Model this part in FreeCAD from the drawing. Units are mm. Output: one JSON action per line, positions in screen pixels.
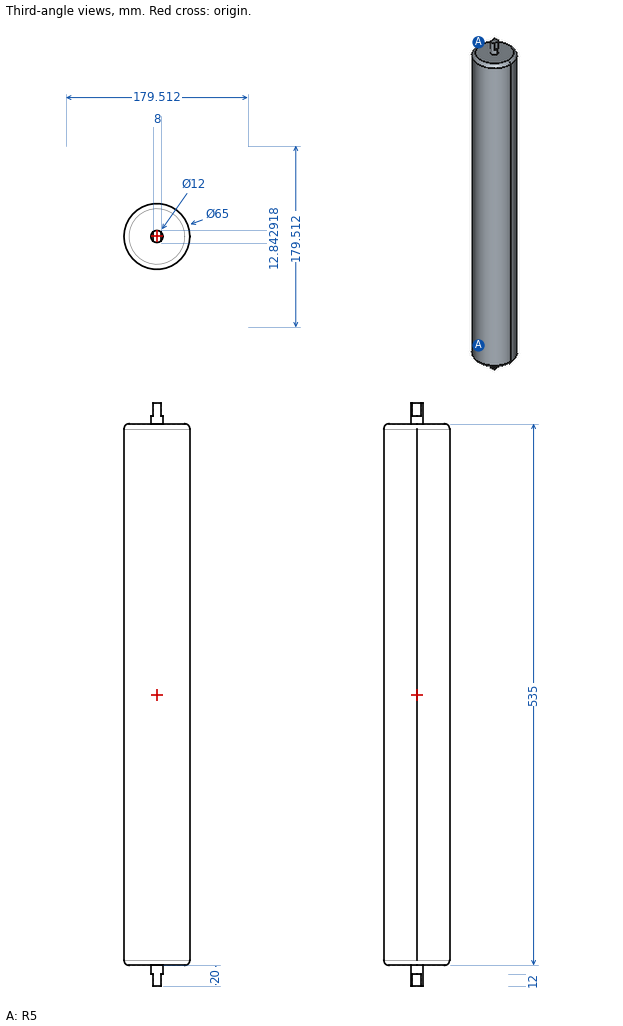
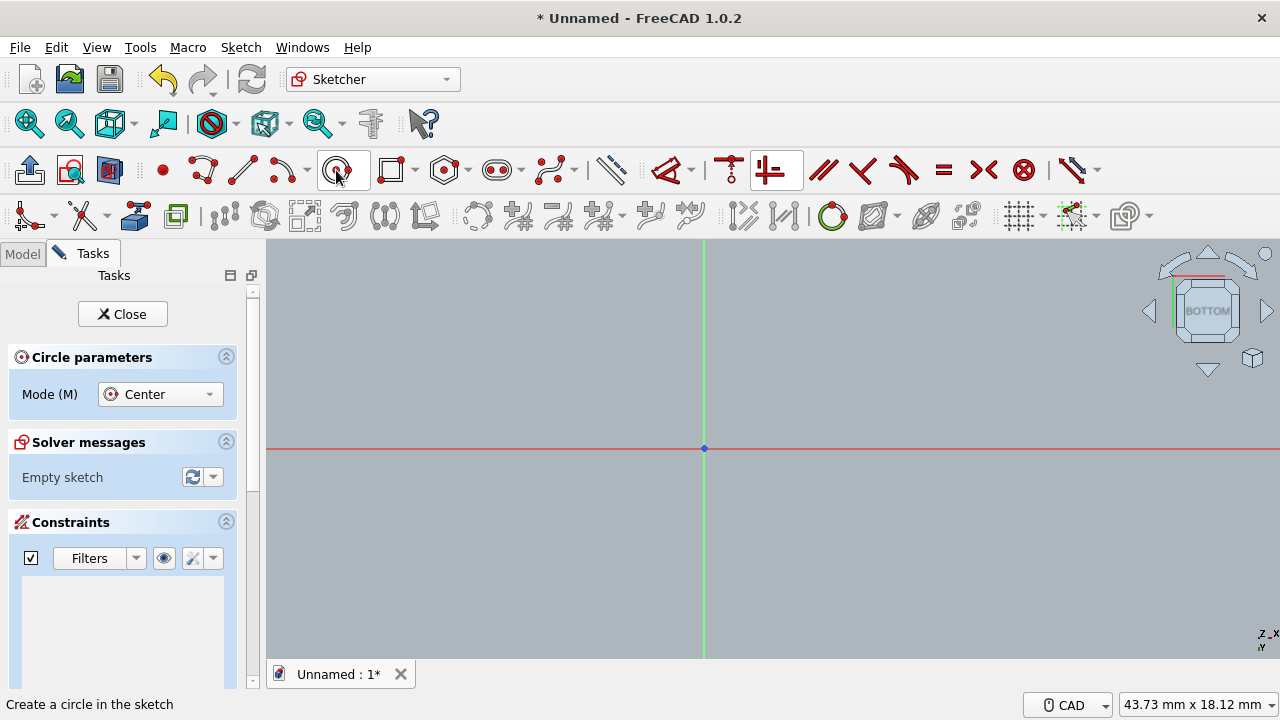
{"action": "left_click", "coordinate": [704, 449]}
{"action": "left_click", "coordinate": [803, 350]}
{"action": "key", "text": "Escape"}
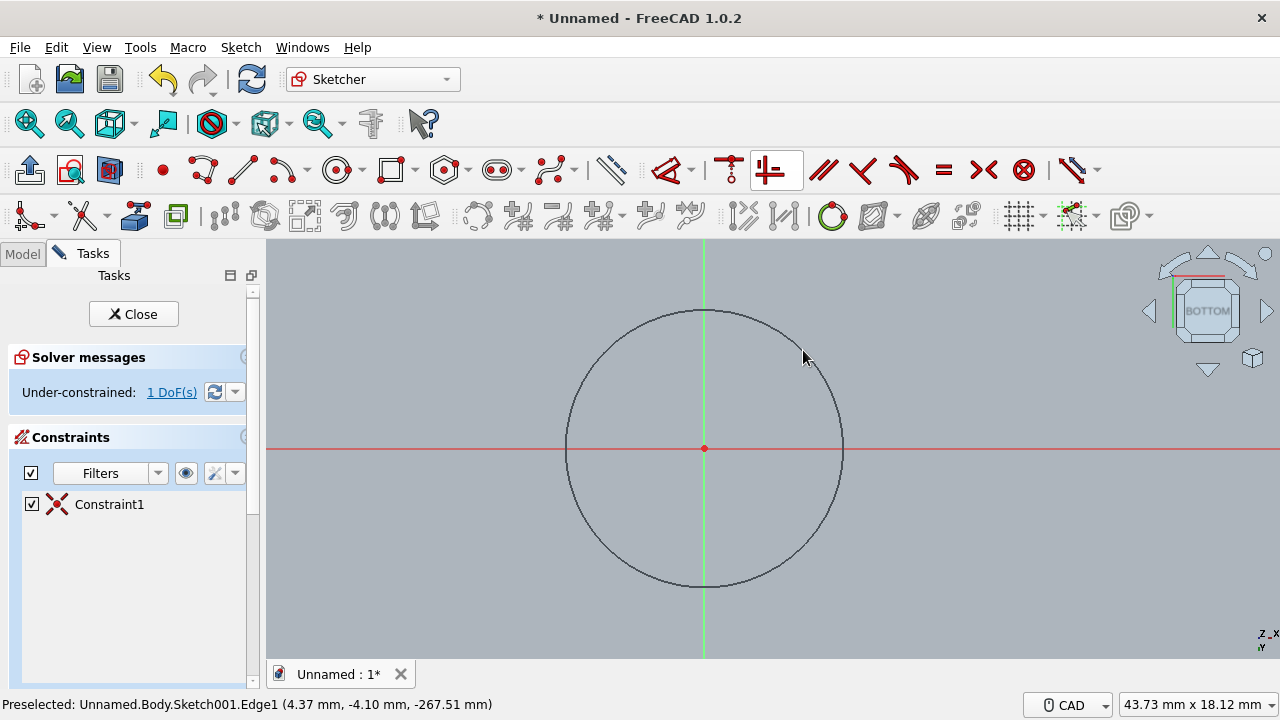
{"action": "left_click", "coordinate": [802, 350]}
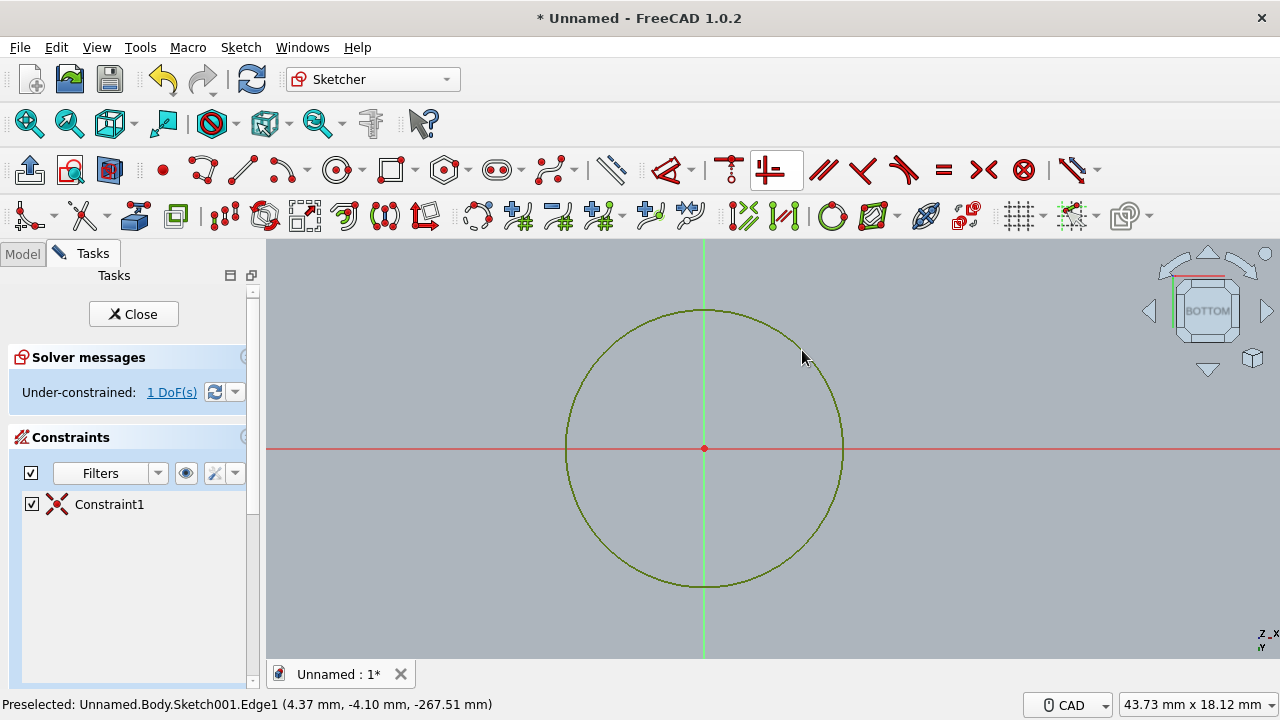
{"action": "left_click", "coordinate": [694, 170]}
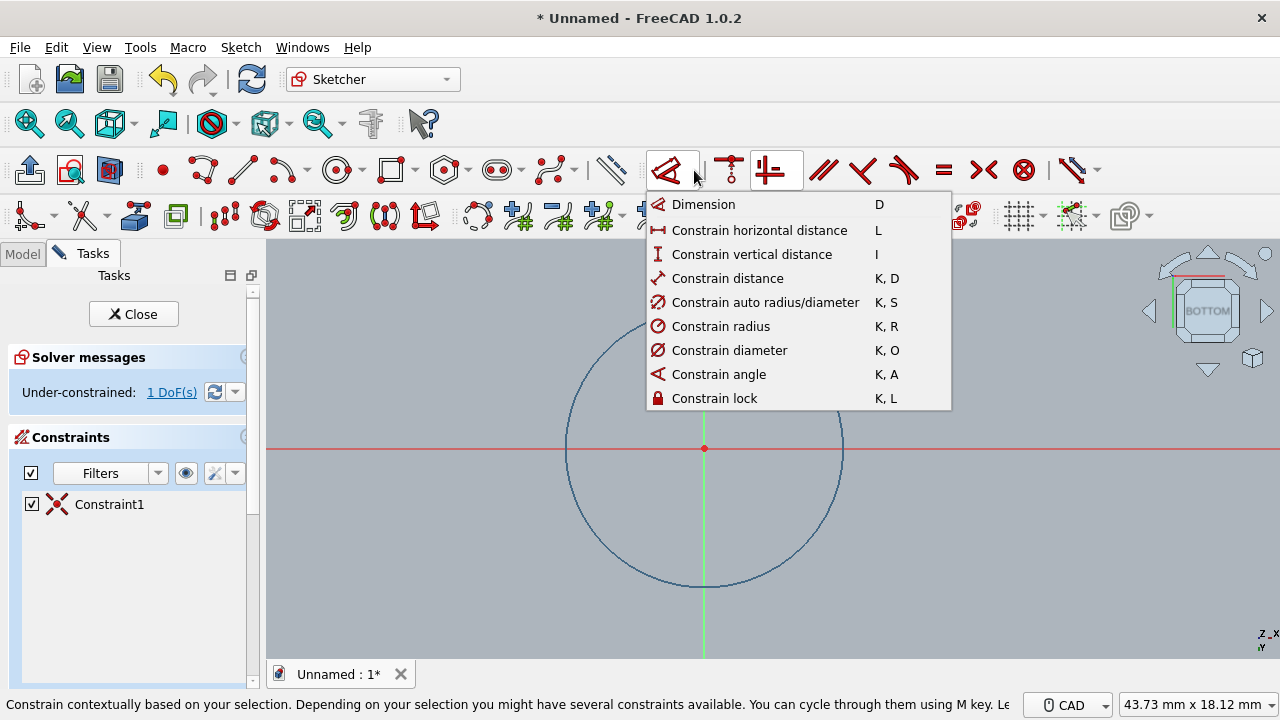
{"action": "left_click", "coordinate": [799, 350]}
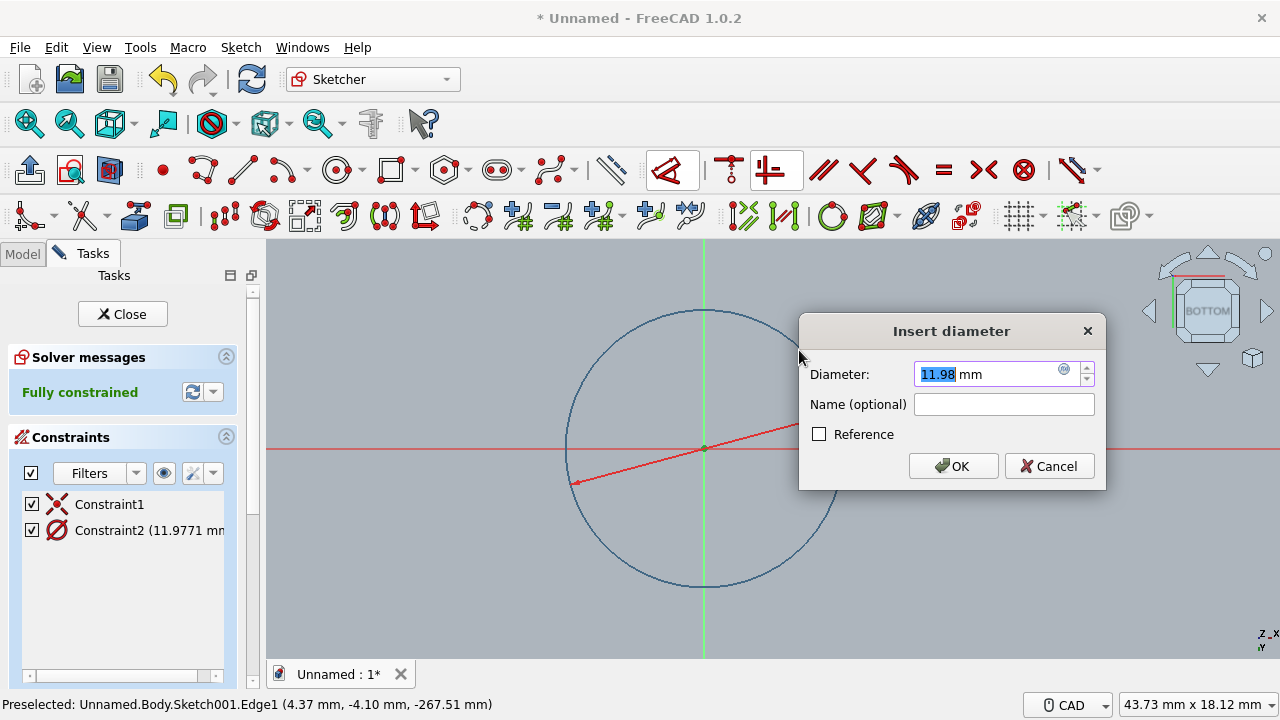
{"action": "type", "text": "12"}
{"action": "key", "text": "Return"}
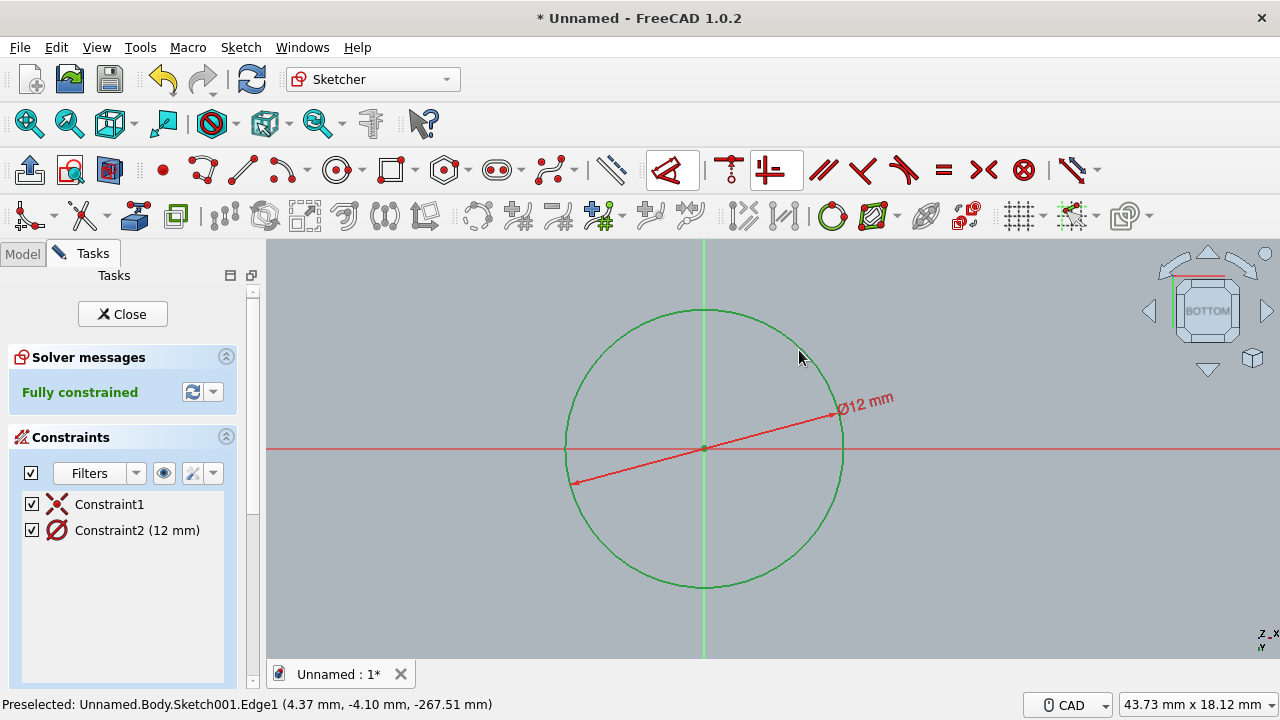
{"action": "left_click", "coordinate": [123, 314]}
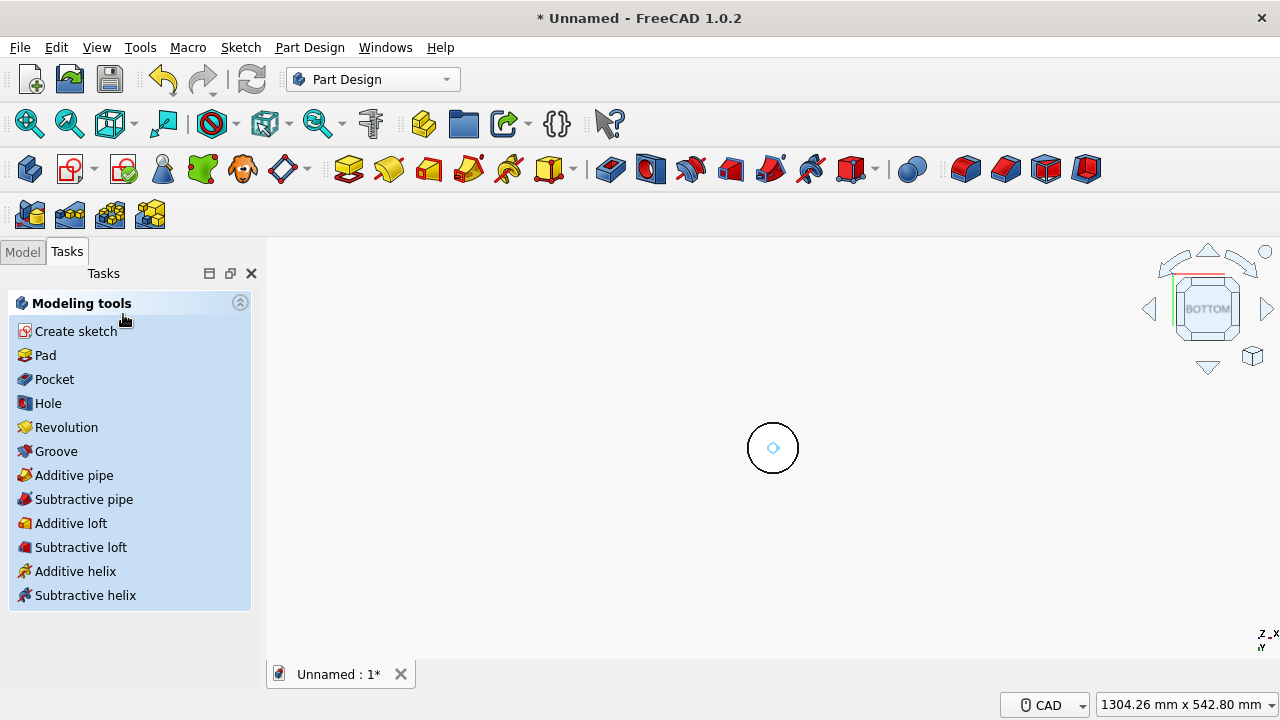
{"action": "left_click", "coordinate": [350, 170]}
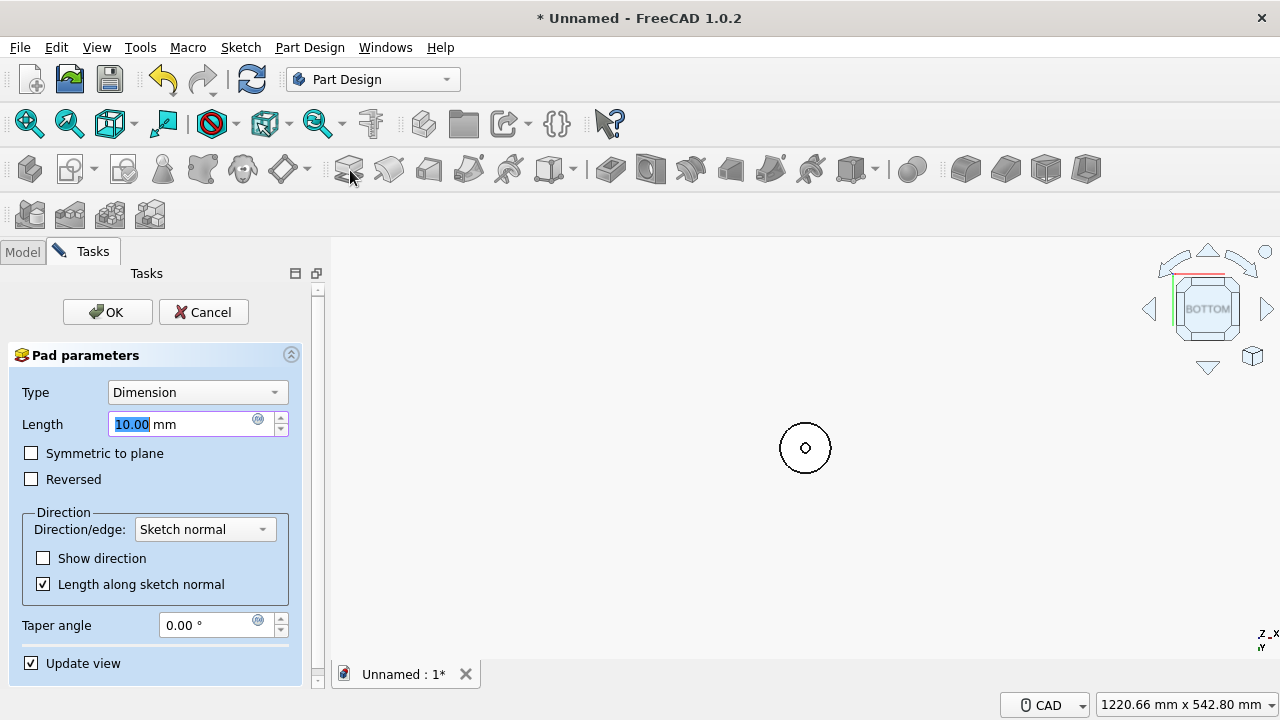
{"action": "type", "text": "20"}
{"action": "key", "text": "Tab"}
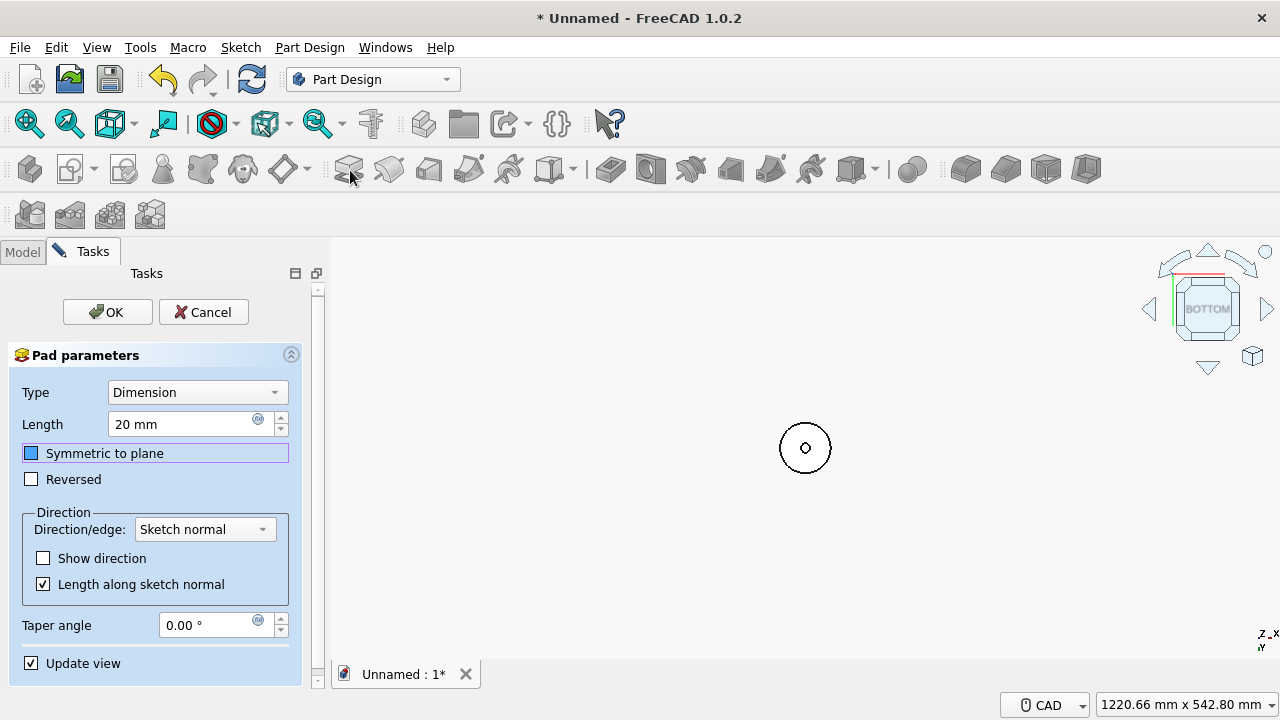
{"action": "left_click", "coordinate": [108, 312]}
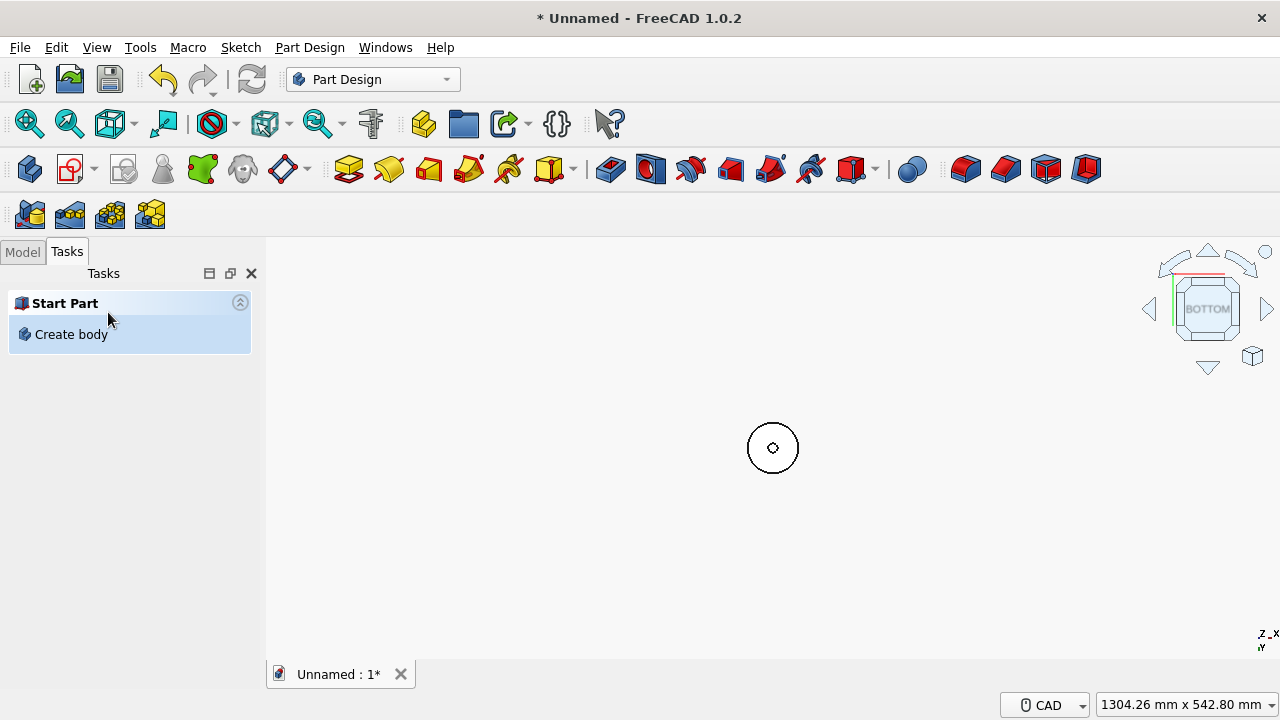
{"action": "left_click", "coordinate": [30, 124]}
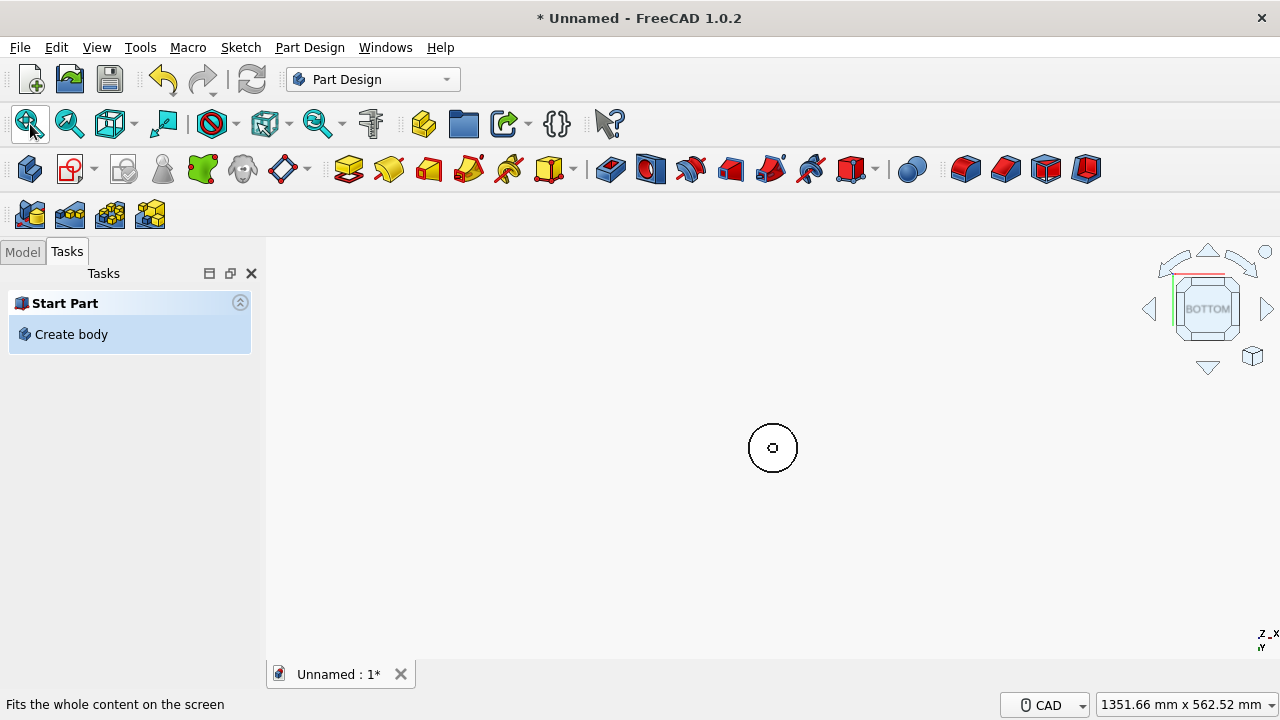
{"action": "scroll", "coordinate": [773, 447], "scroll_direction": "up", "scroll_amount": 5}